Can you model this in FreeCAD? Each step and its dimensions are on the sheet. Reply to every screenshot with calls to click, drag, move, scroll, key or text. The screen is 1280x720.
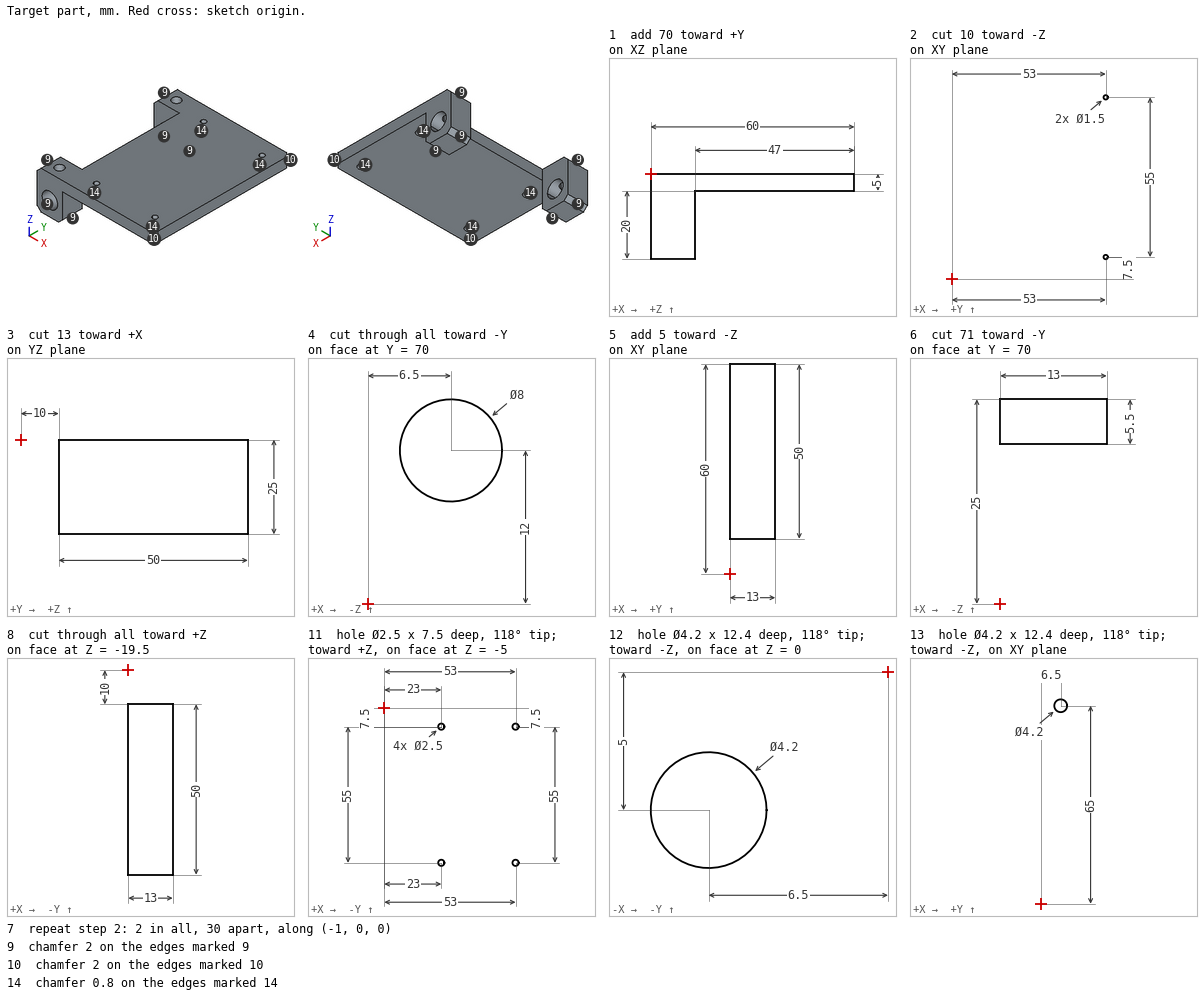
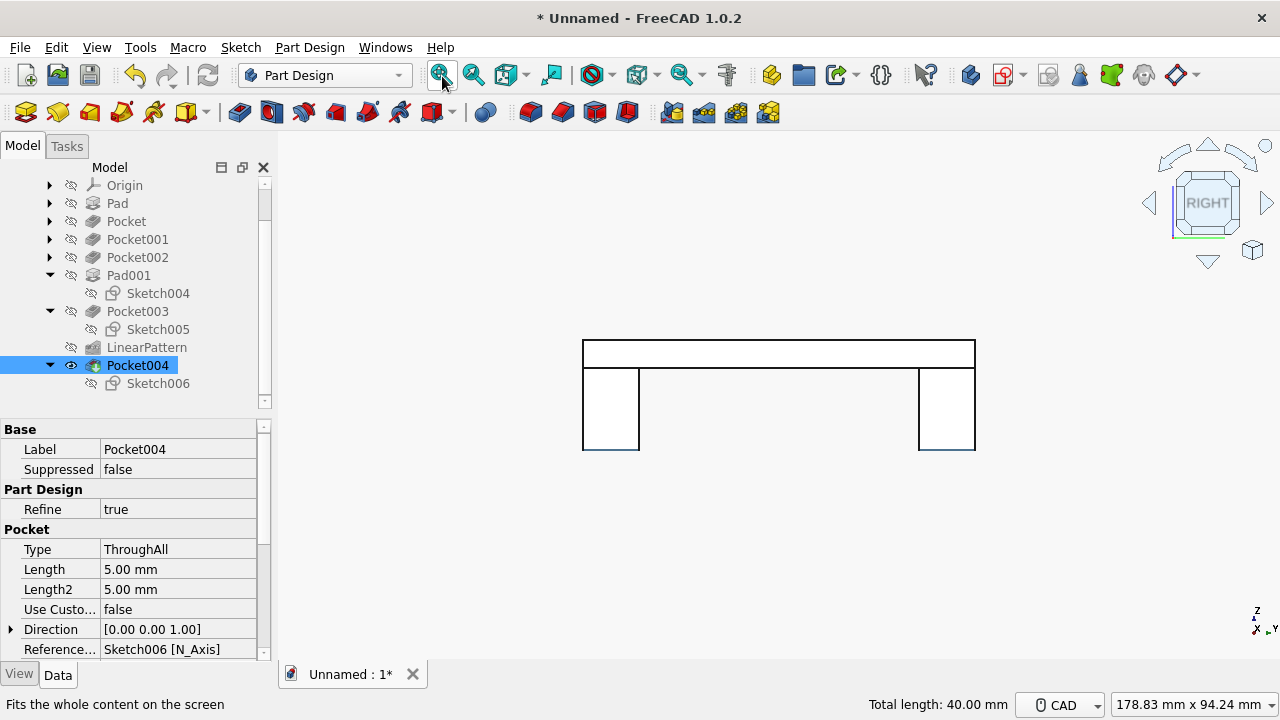
click(442, 76)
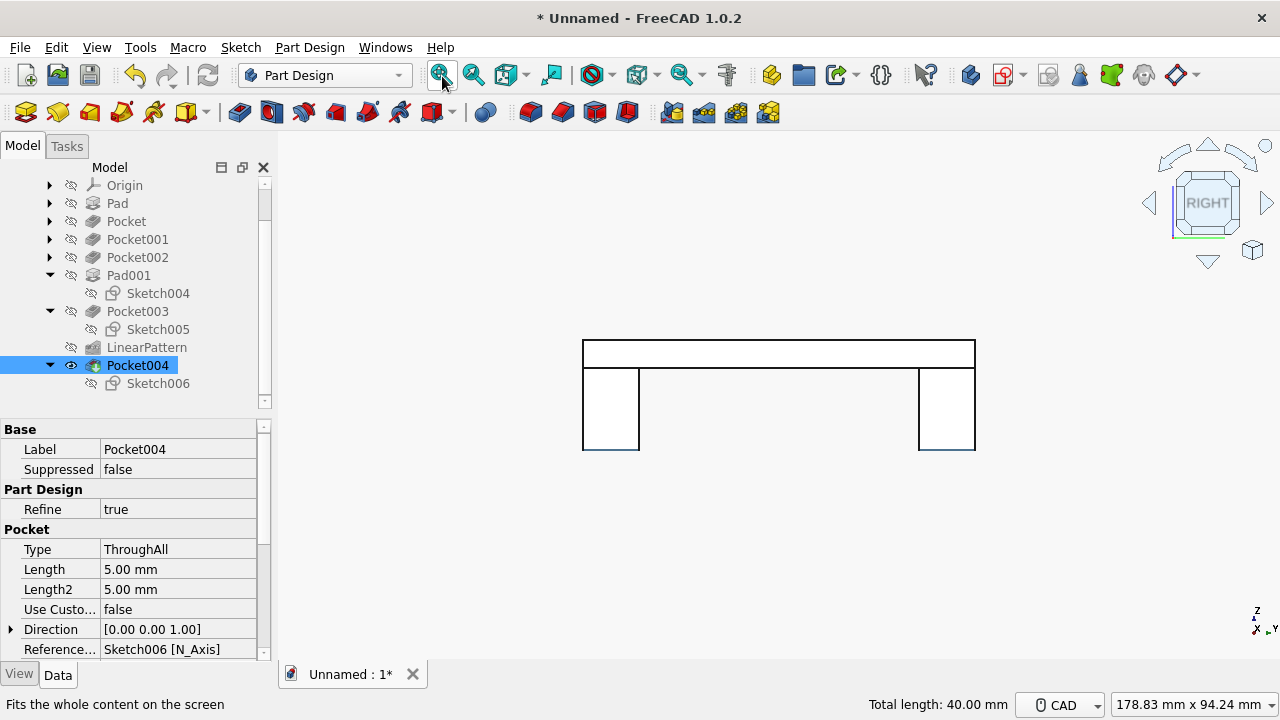
key(5)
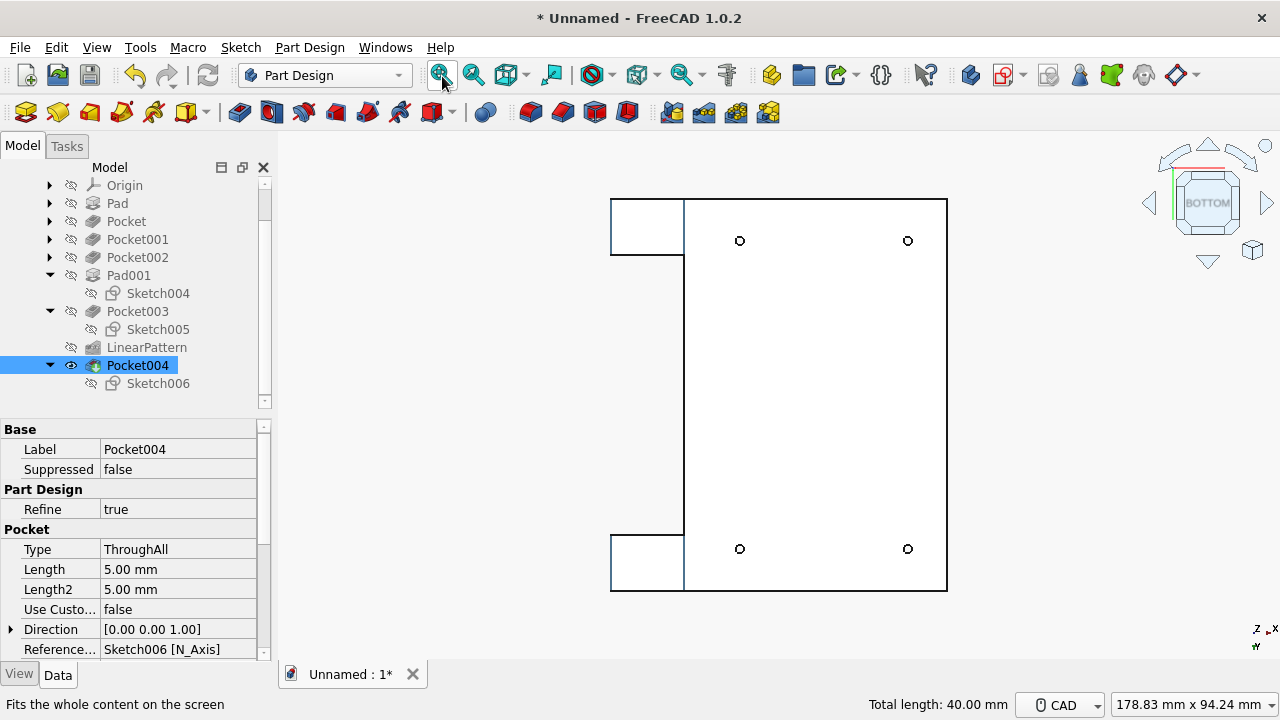
key(4)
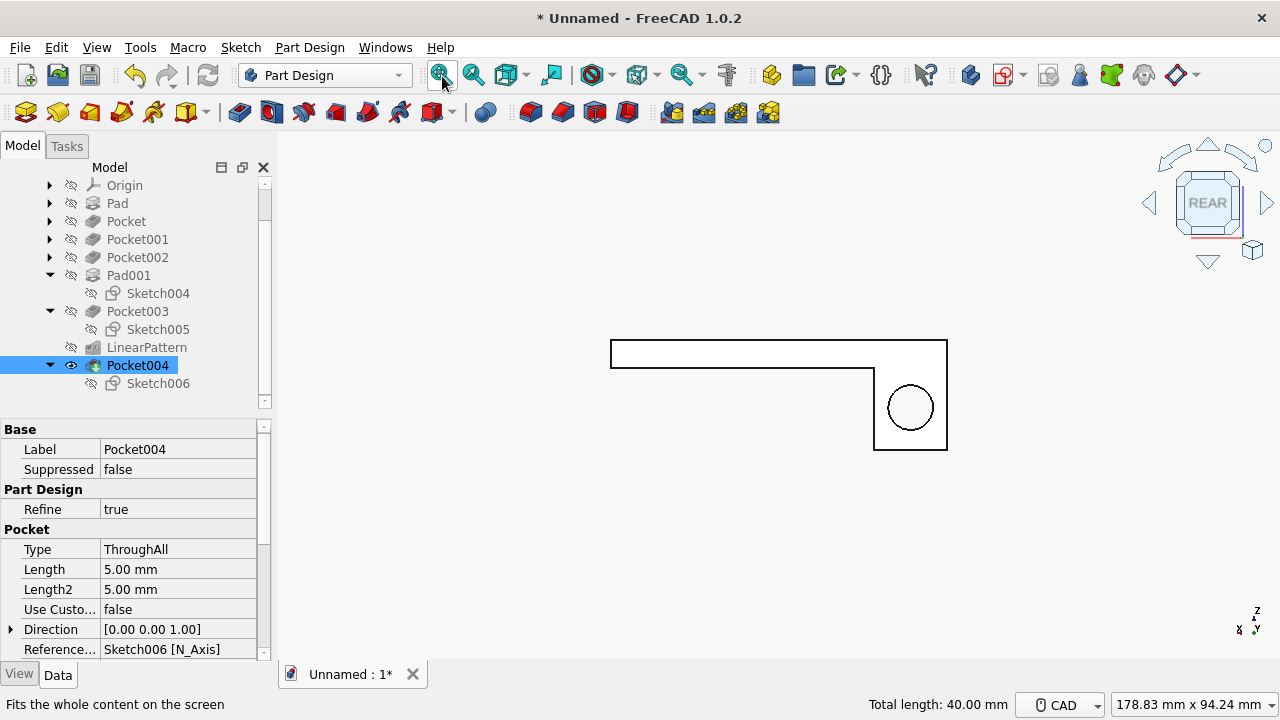
key(v)
key(f)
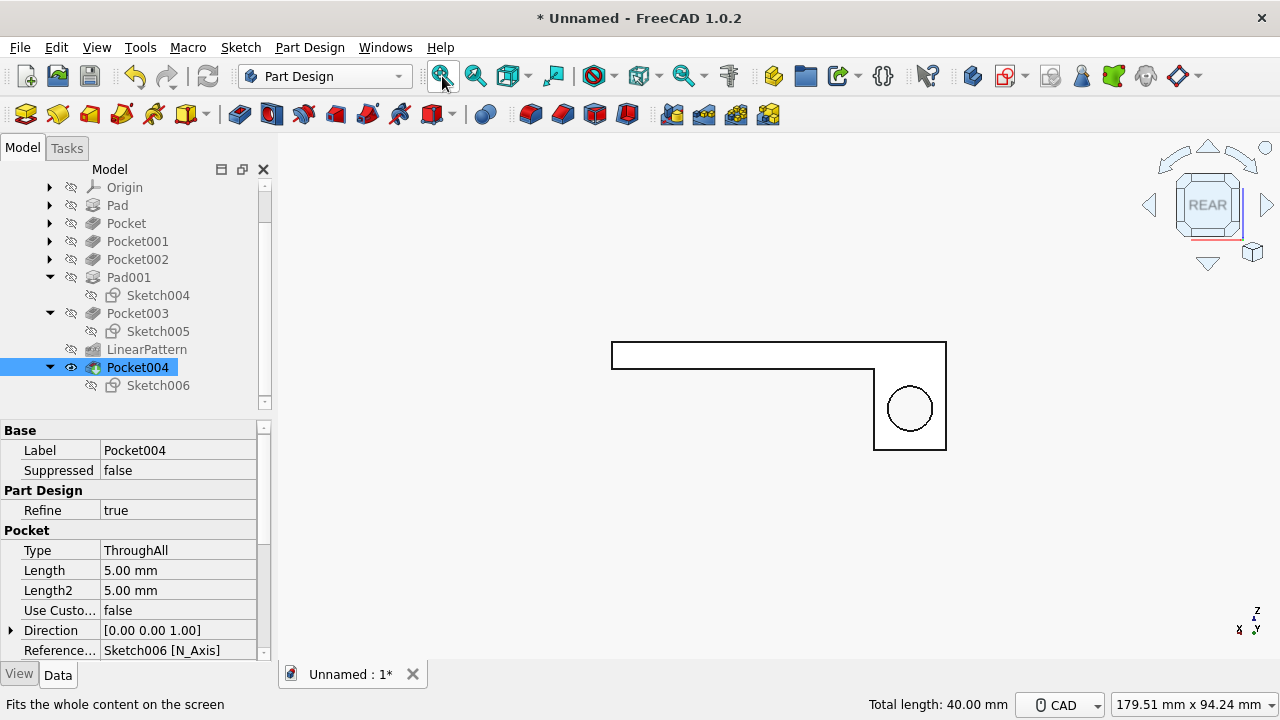
key(6)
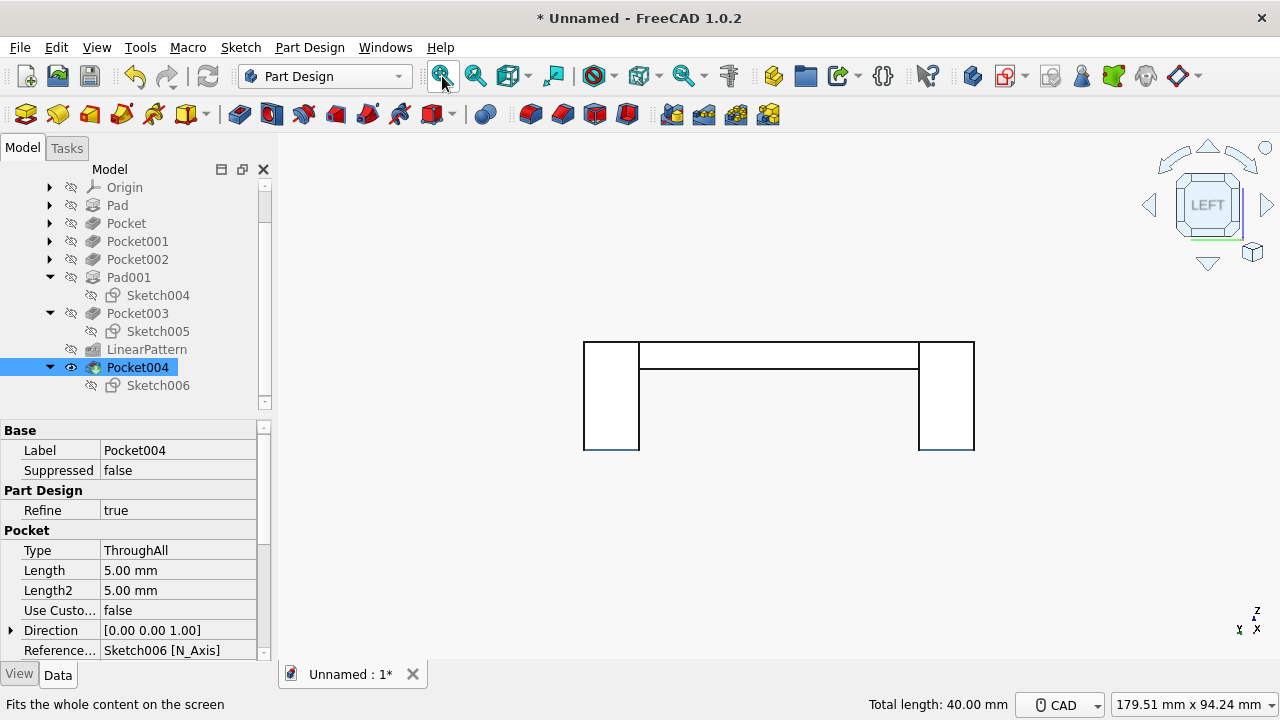
key(v)
key(f)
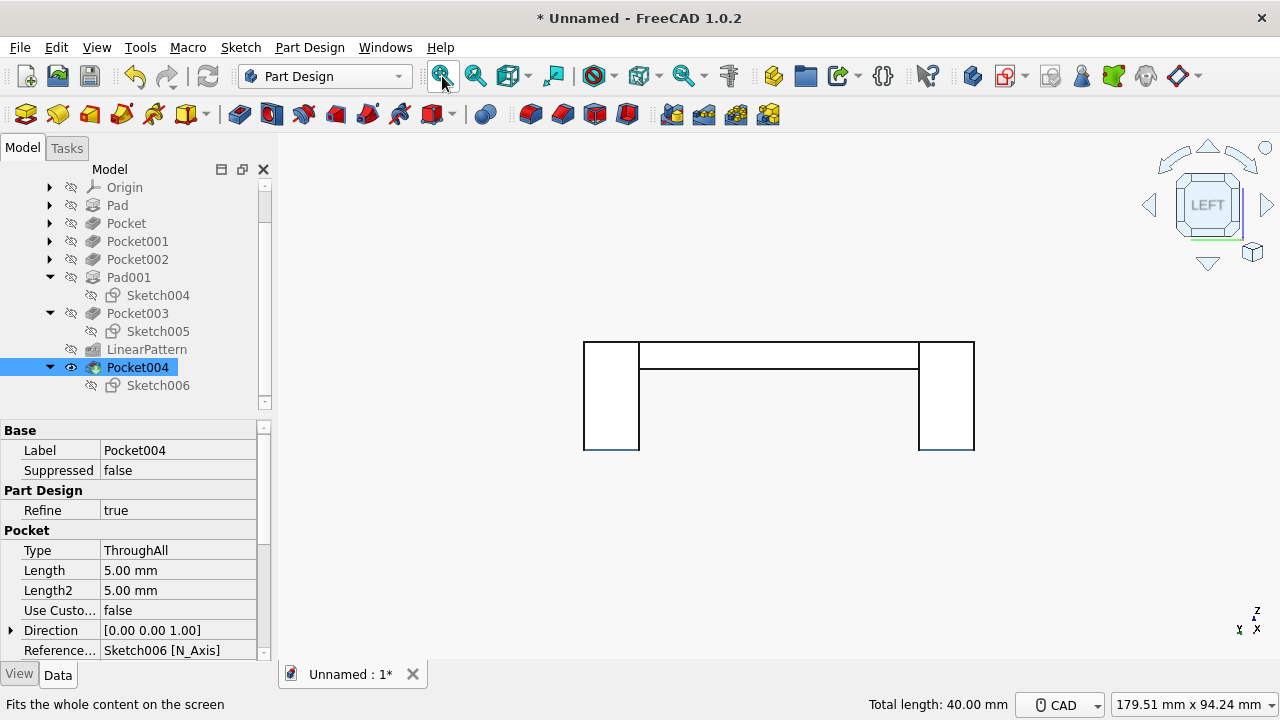
click(612, 341, ctrl)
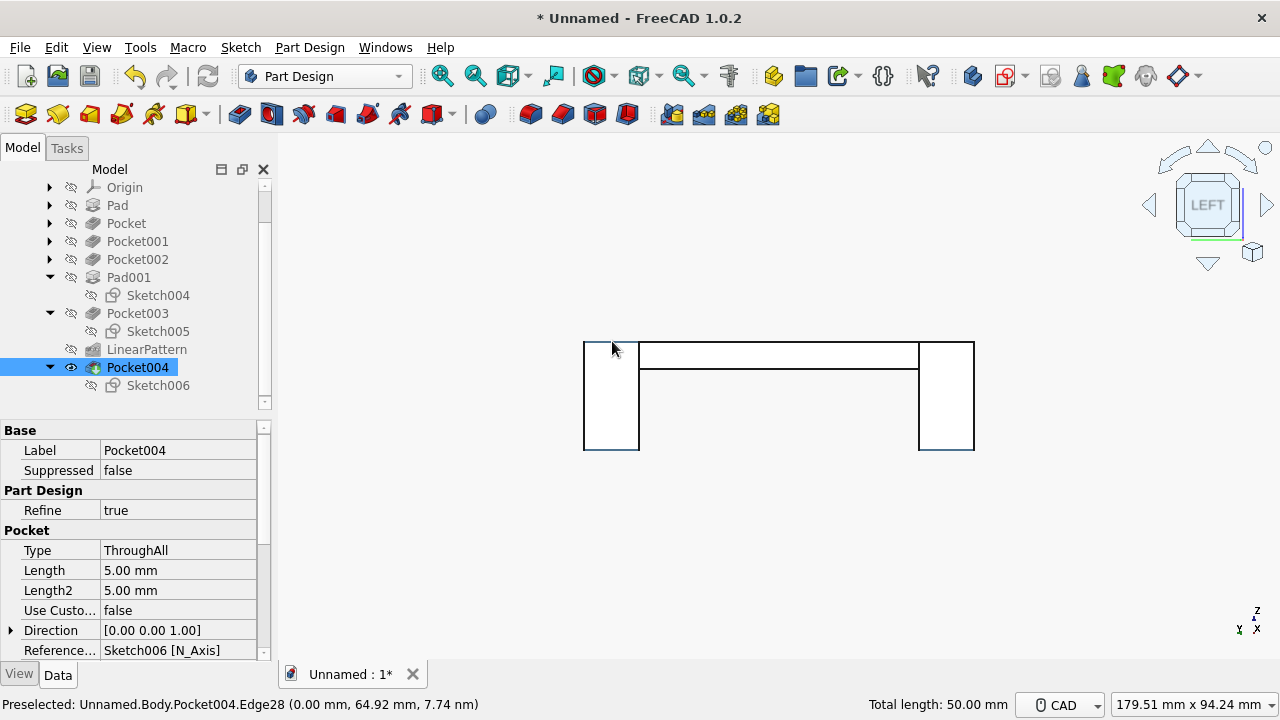
click(946, 341, ctrl)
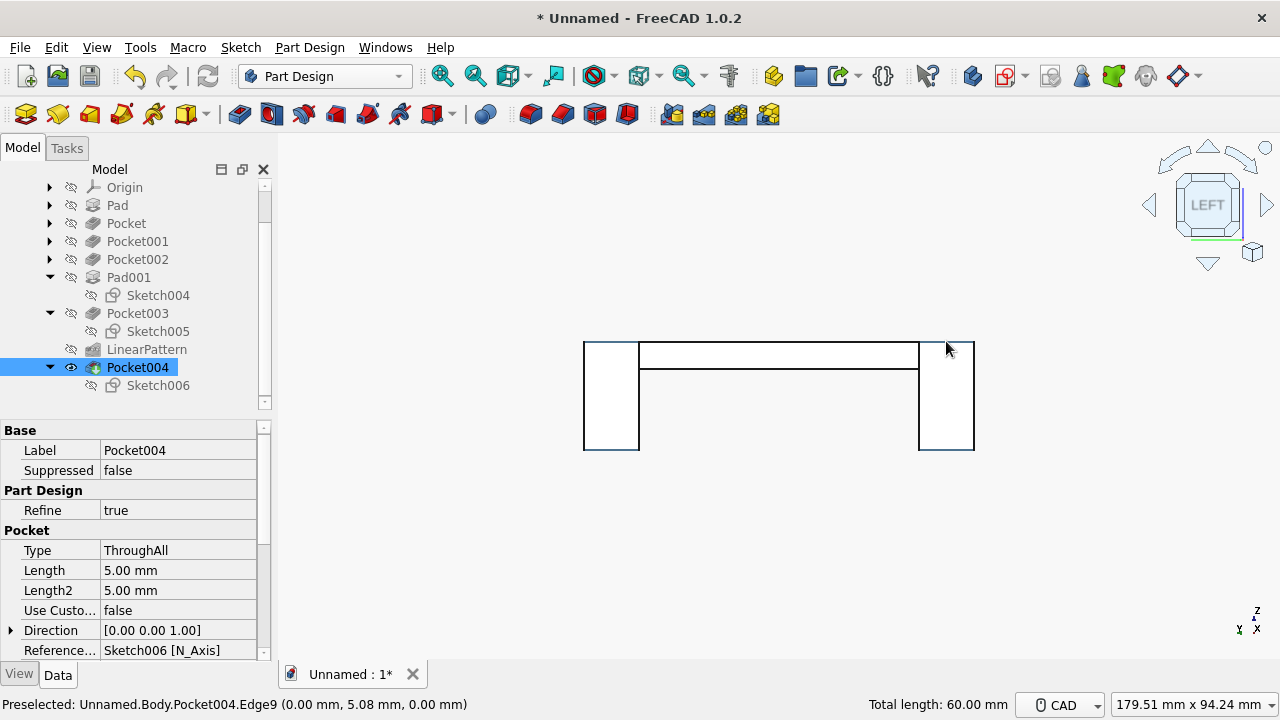
click(564, 114)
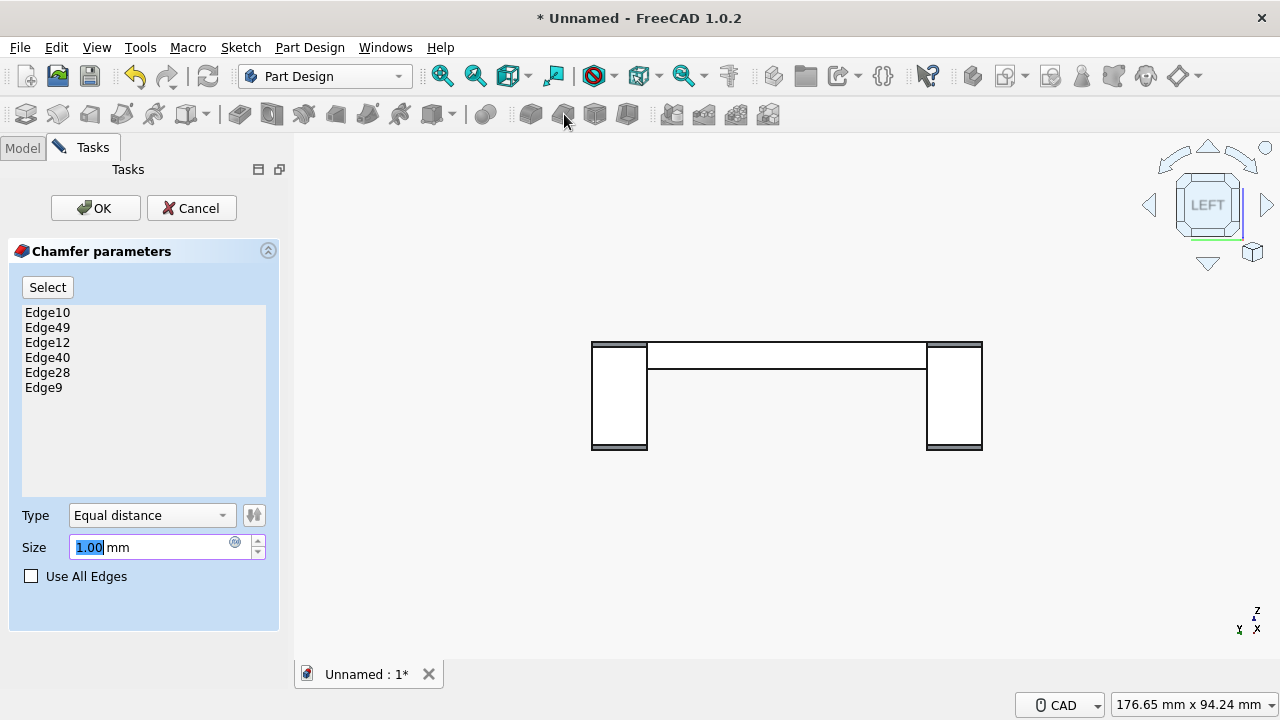
text(2)
key(Tab)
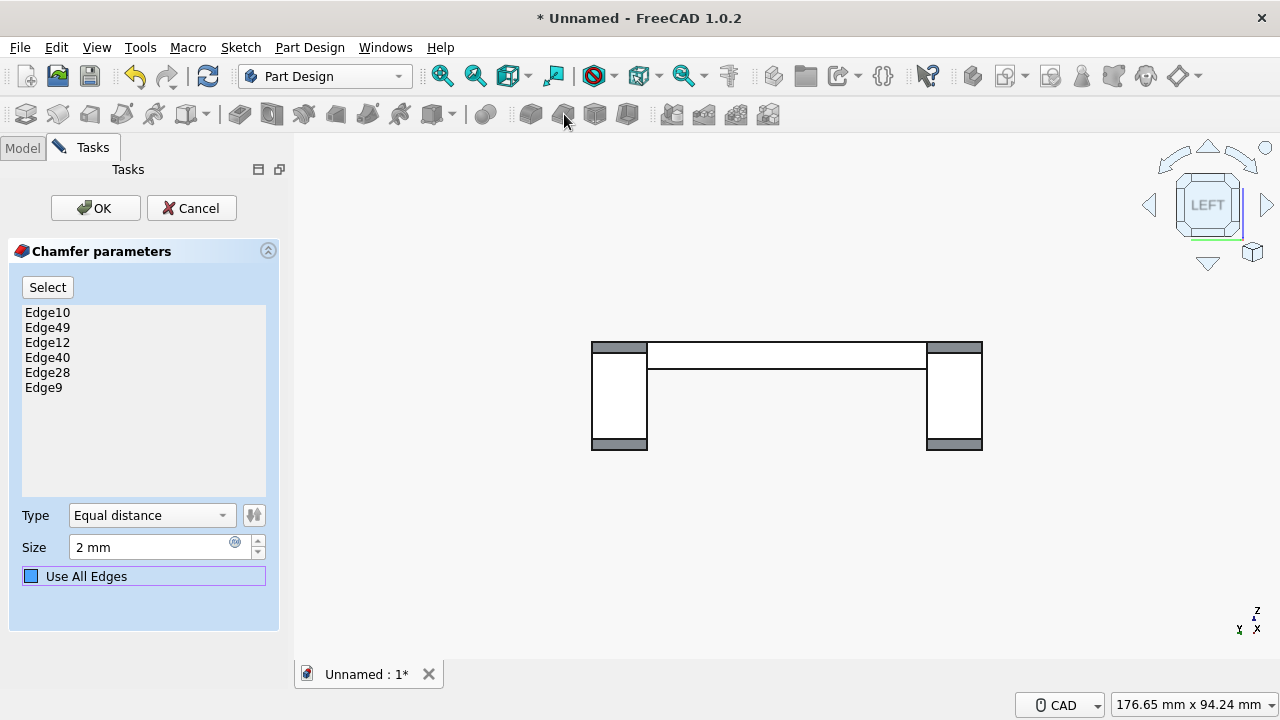
click(96, 208)